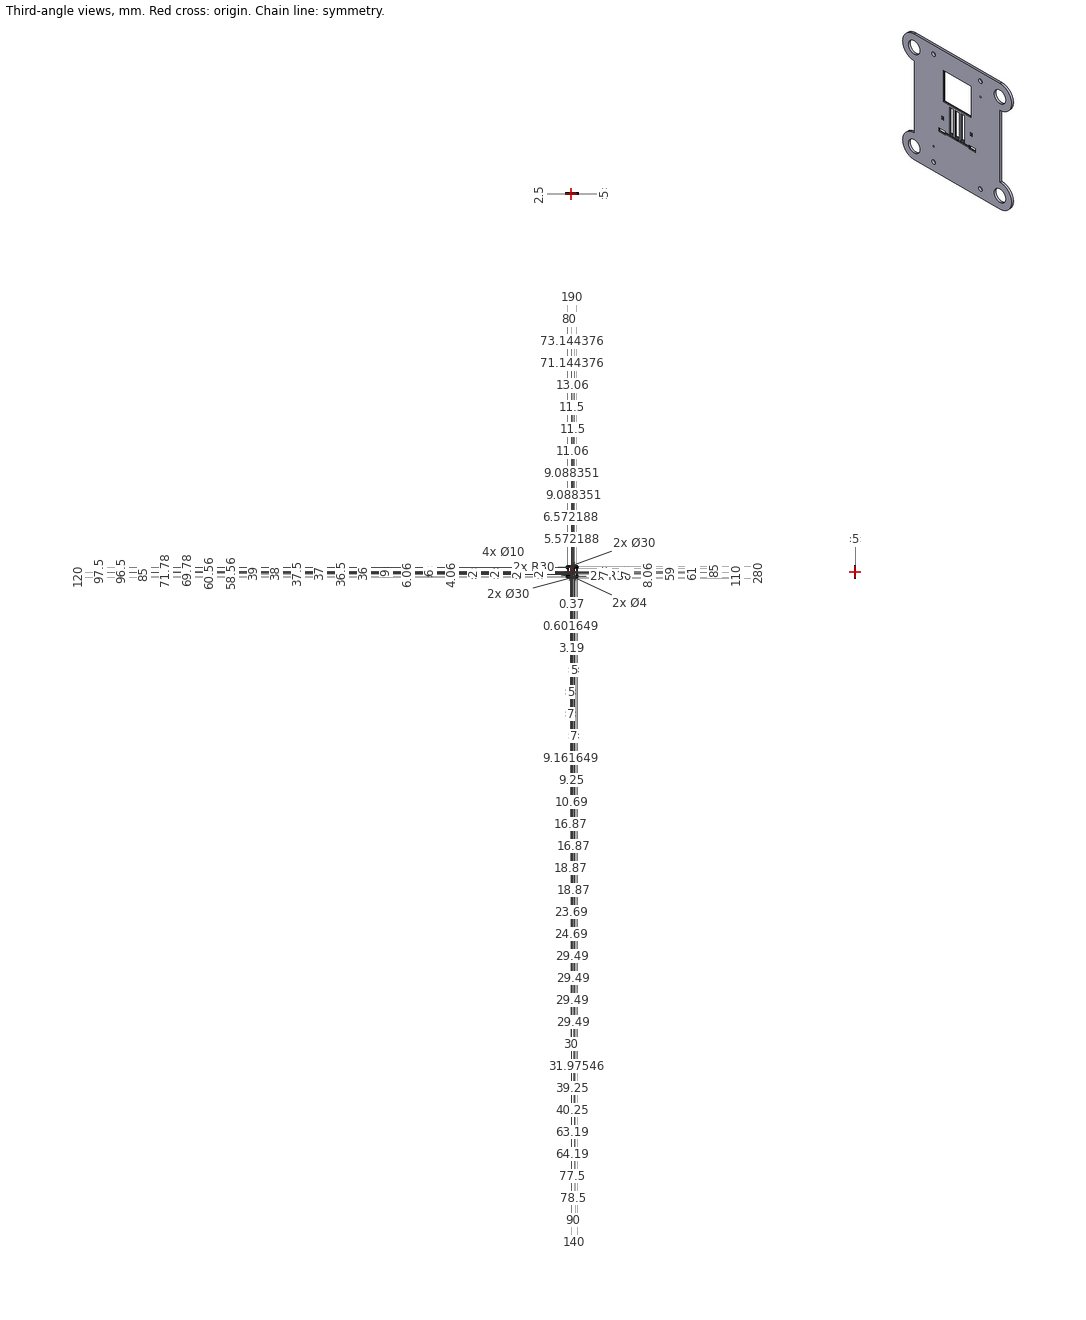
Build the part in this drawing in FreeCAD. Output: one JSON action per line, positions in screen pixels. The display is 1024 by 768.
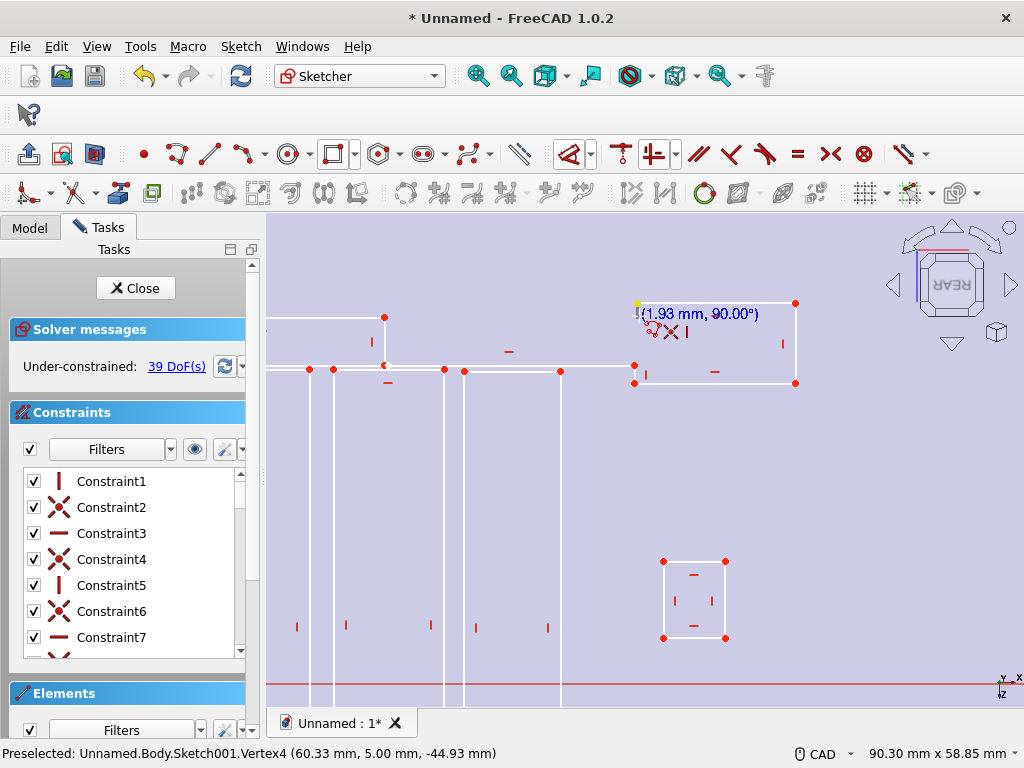
{"action": "left_click", "coordinate": [637, 315]}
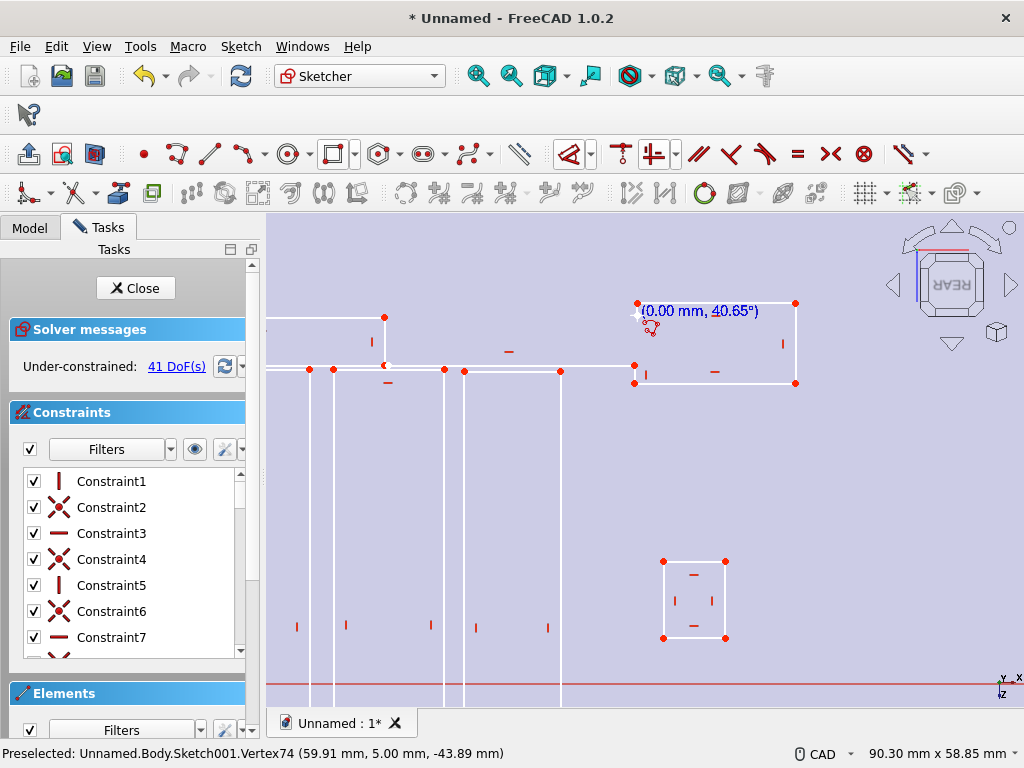
{"action": "scroll", "coordinate": [388, 315], "scroll_direction": "up", "scroll_amount": 10}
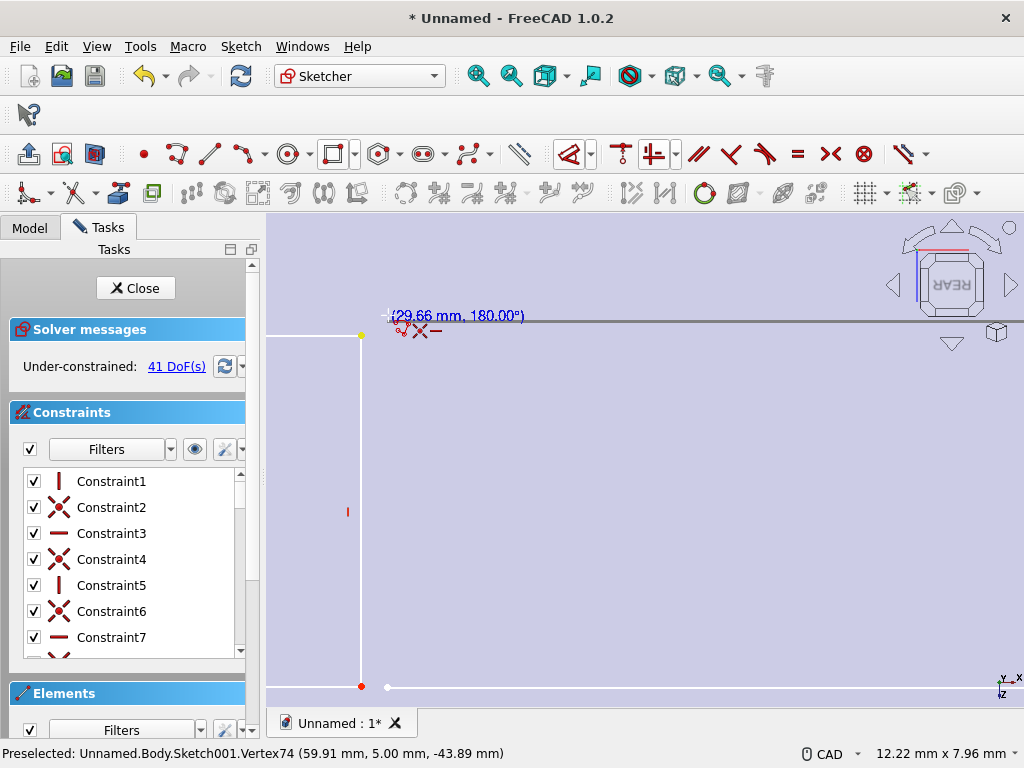
{"action": "left_click", "coordinate": [388, 314]}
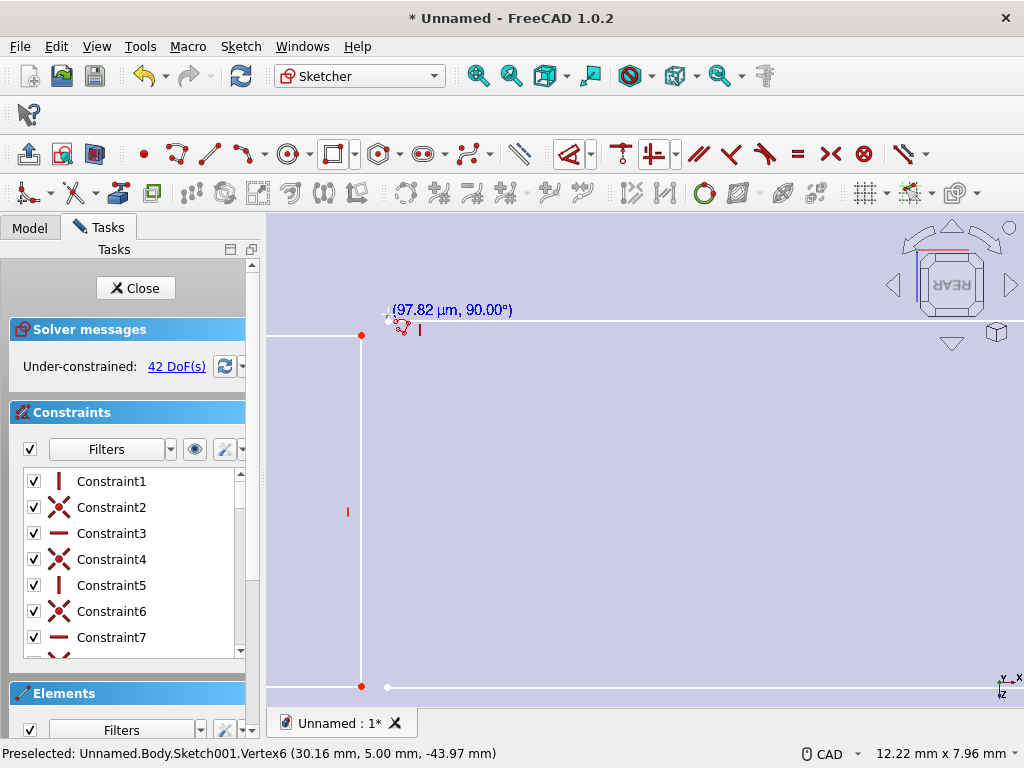
{"action": "scroll", "coordinate": [585, 282], "scroll_direction": "down", "scroll_amount": 16}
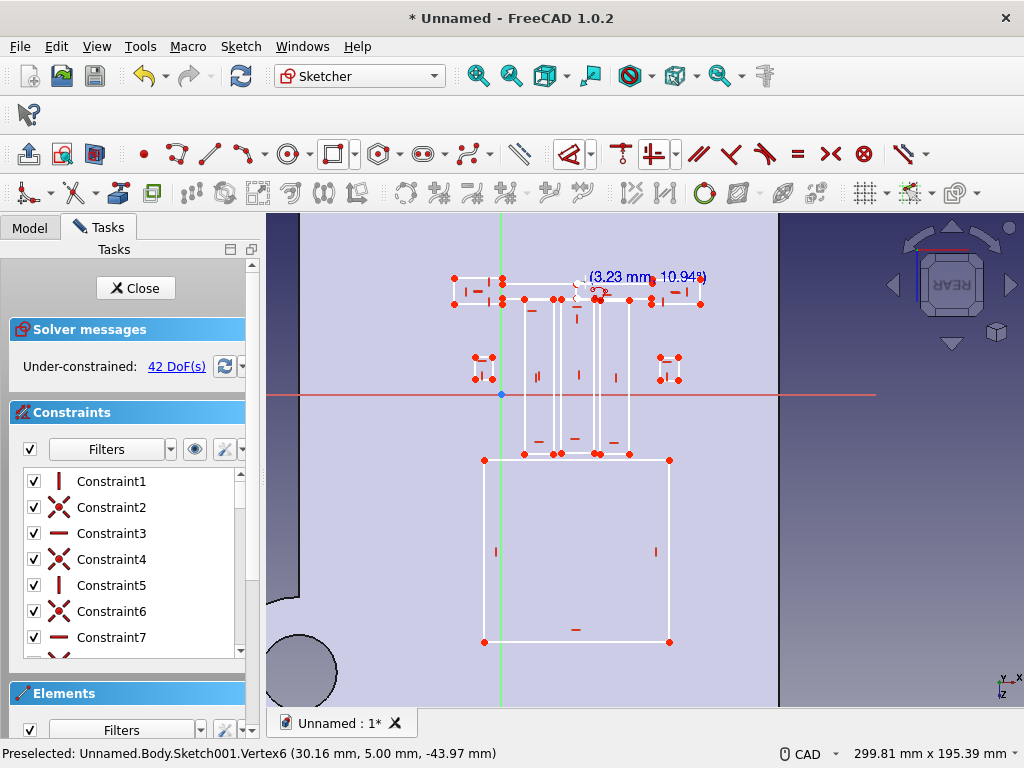
{"action": "scroll", "coordinate": [577, 299], "scroll_direction": "up", "scroll_amount": 16}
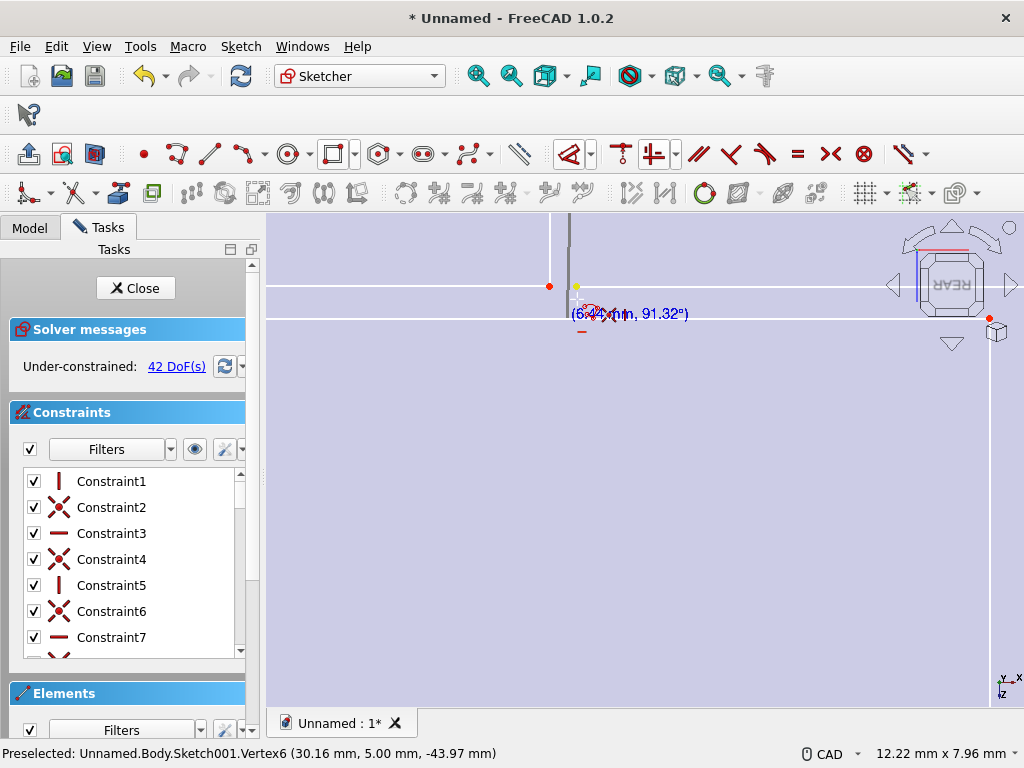
{"action": "left_click", "coordinate": [576, 287]}
{"action": "key", "text": "Escape"}
{"action": "key", "text": "Escape"}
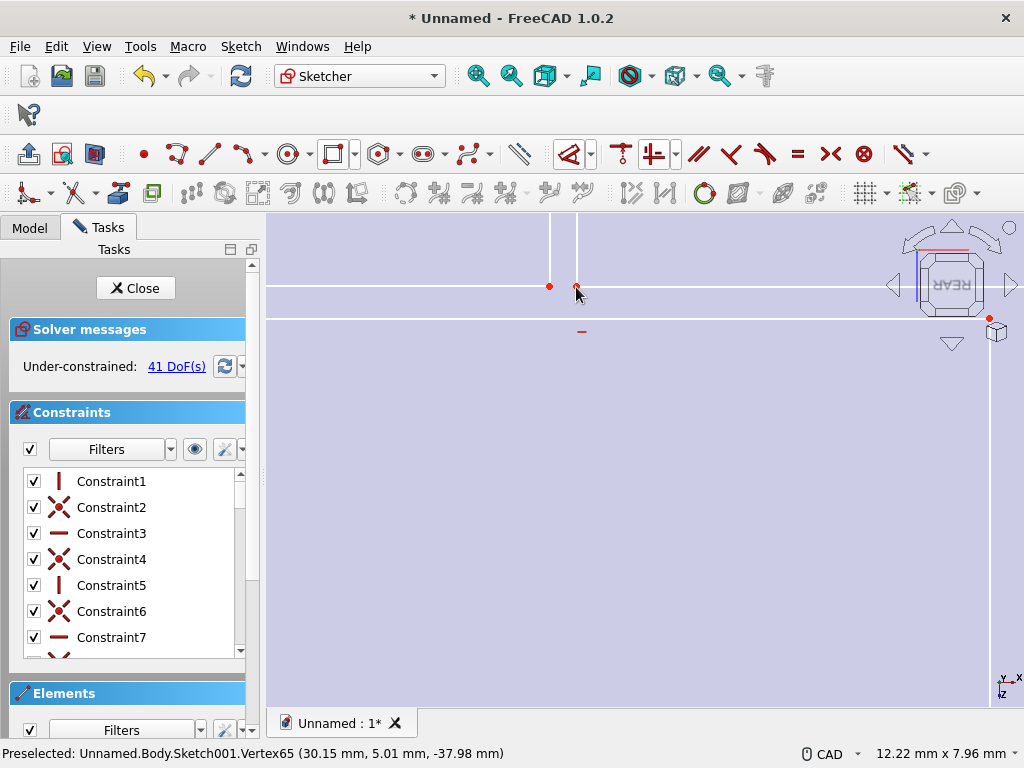
{"action": "scroll", "coordinate": [577, 299], "scroll_direction": "down", "scroll_amount": 16}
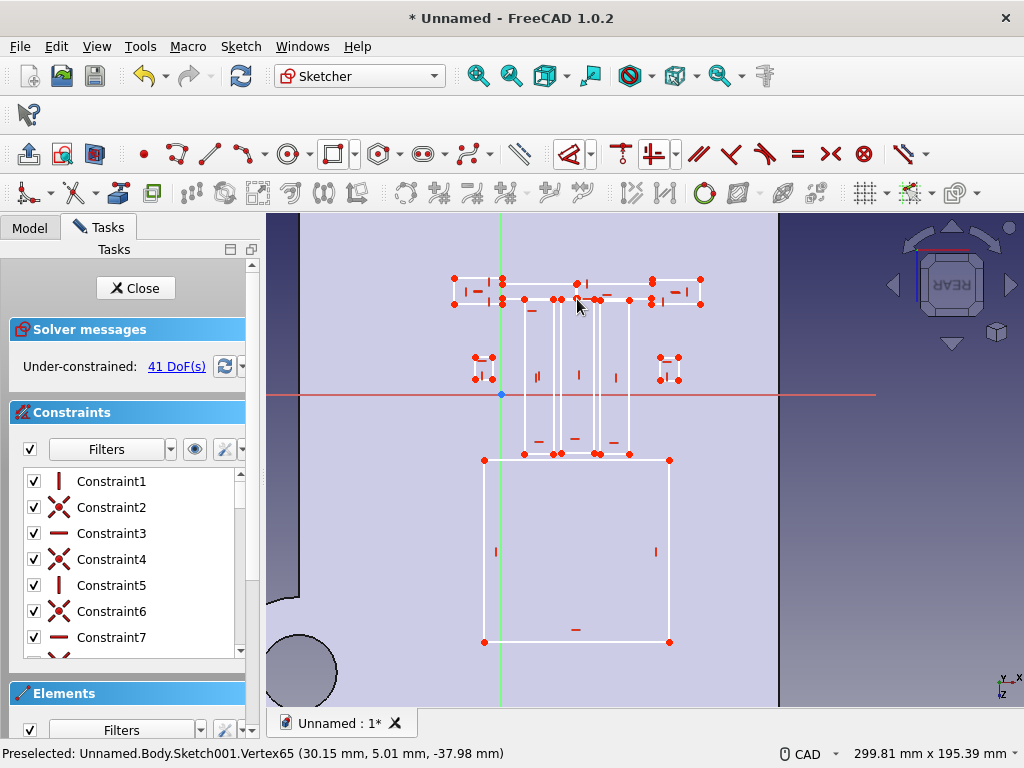
{"action": "scroll", "coordinate": [652, 281], "scroll_direction": "up", "scroll_amount": 13}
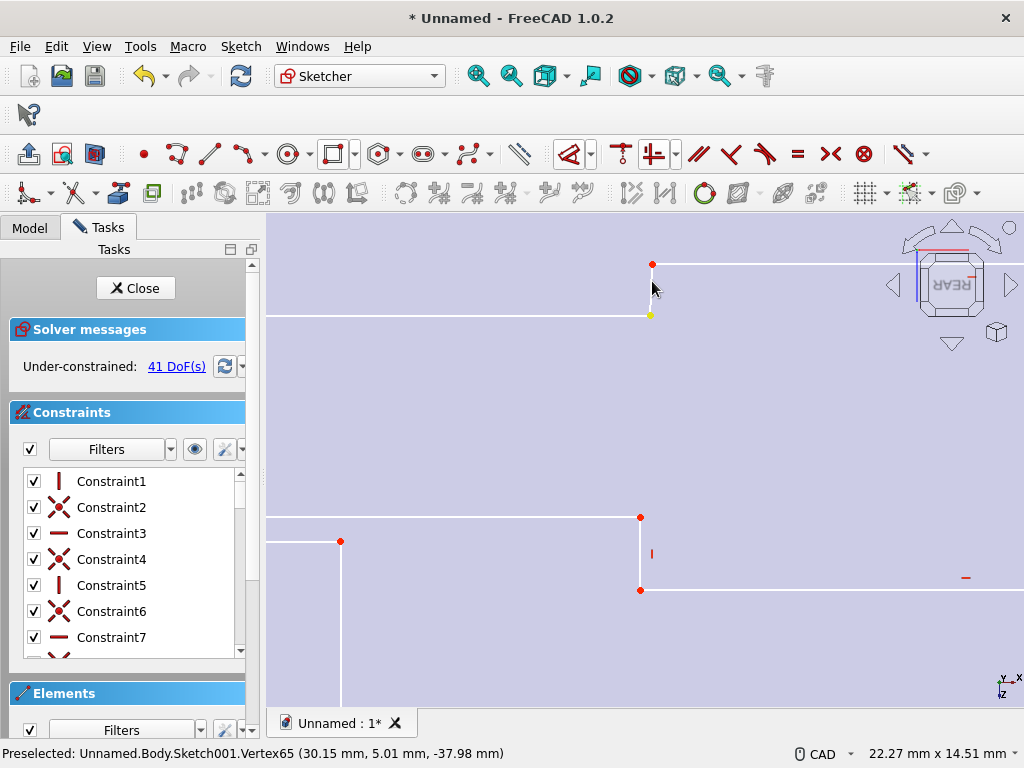
{"action": "left_click", "coordinate": [651, 280]}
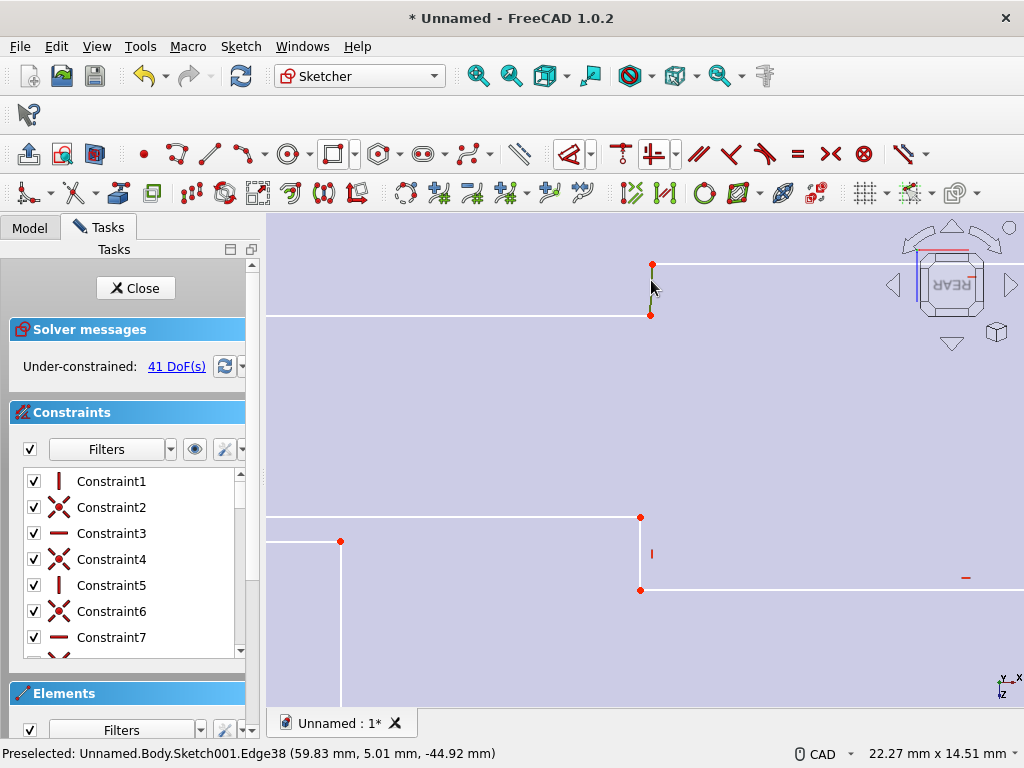
{"action": "left_click", "coordinate": [676, 154]}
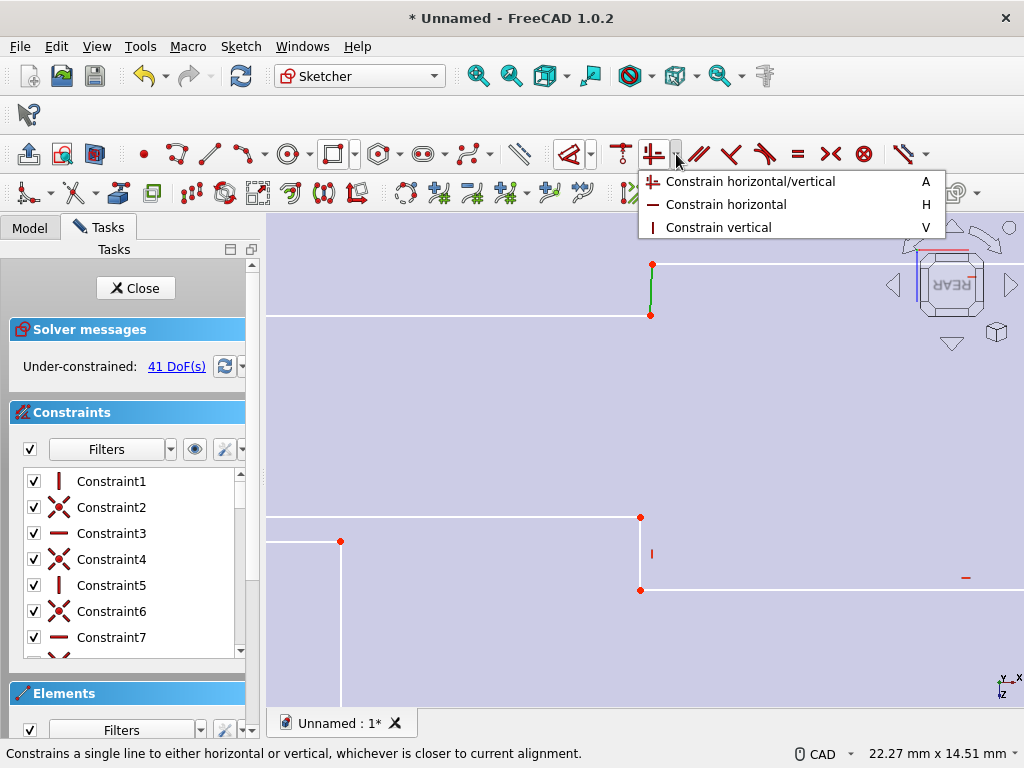
{"action": "left_click", "coordinate": [792, 228]}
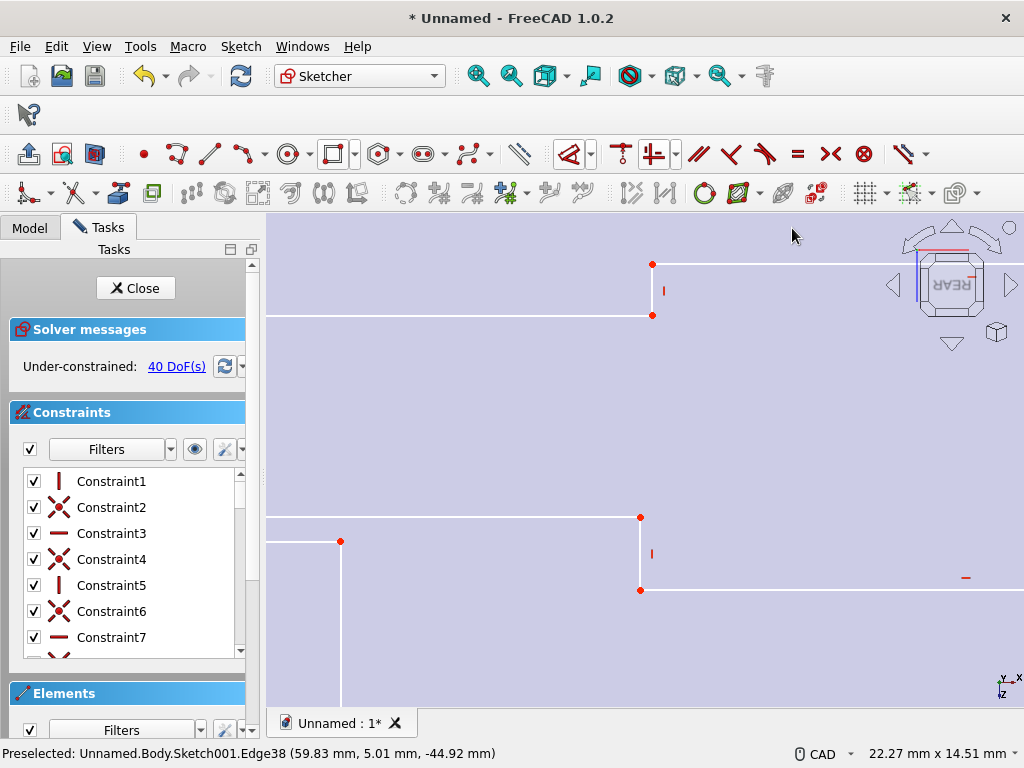
{"action": "scroll", "coordinate": [637, 316], "scroll_direction": "down", "scroll_amount": 14}